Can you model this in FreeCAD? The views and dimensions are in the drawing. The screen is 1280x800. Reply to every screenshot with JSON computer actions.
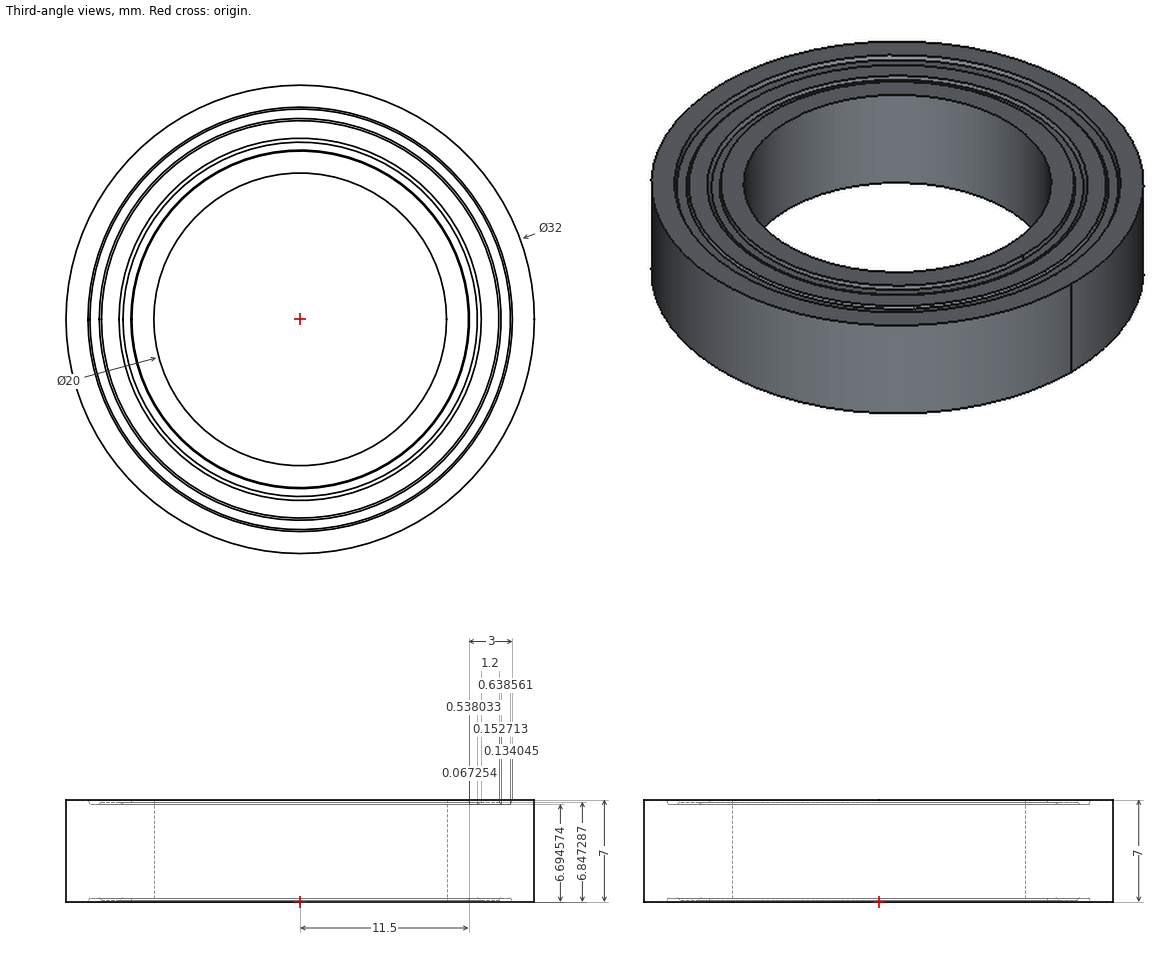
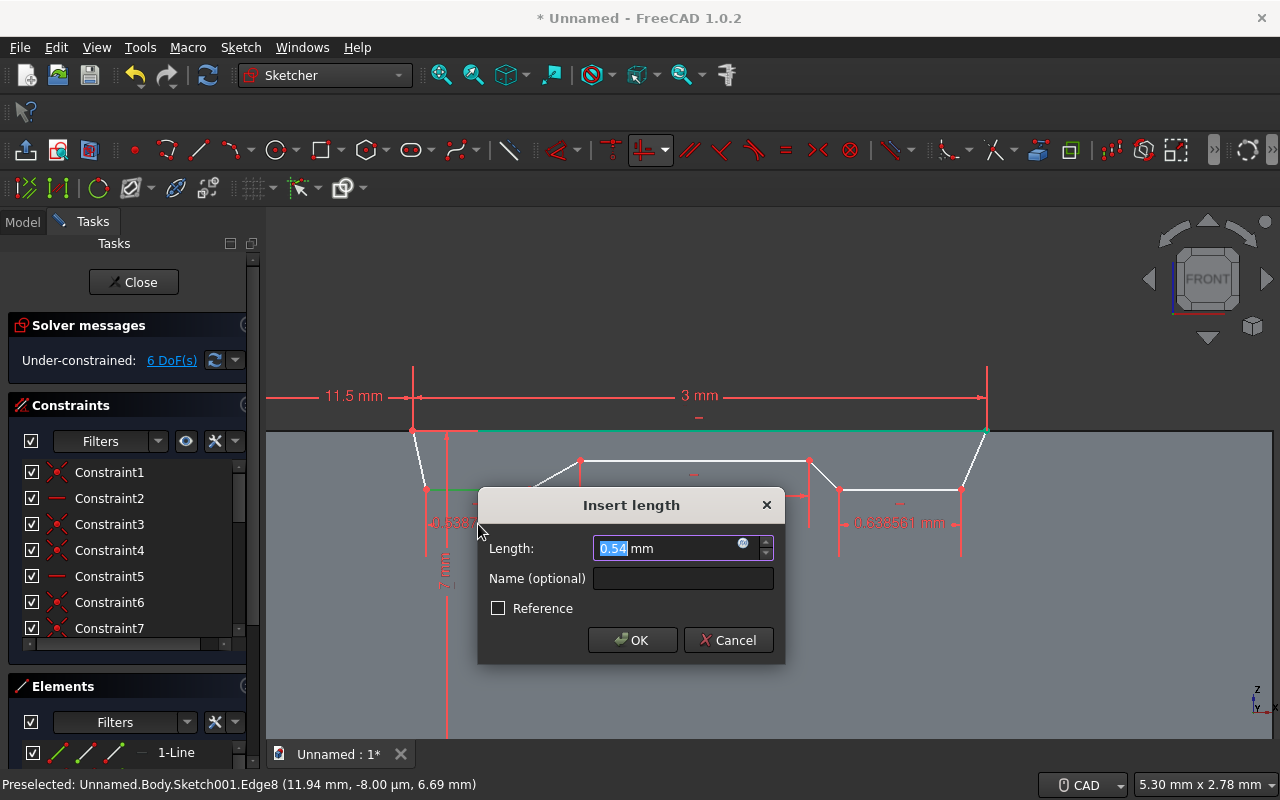
{"action": "type", "text": "0.538033"}
{"action": "key", "text": "Return"}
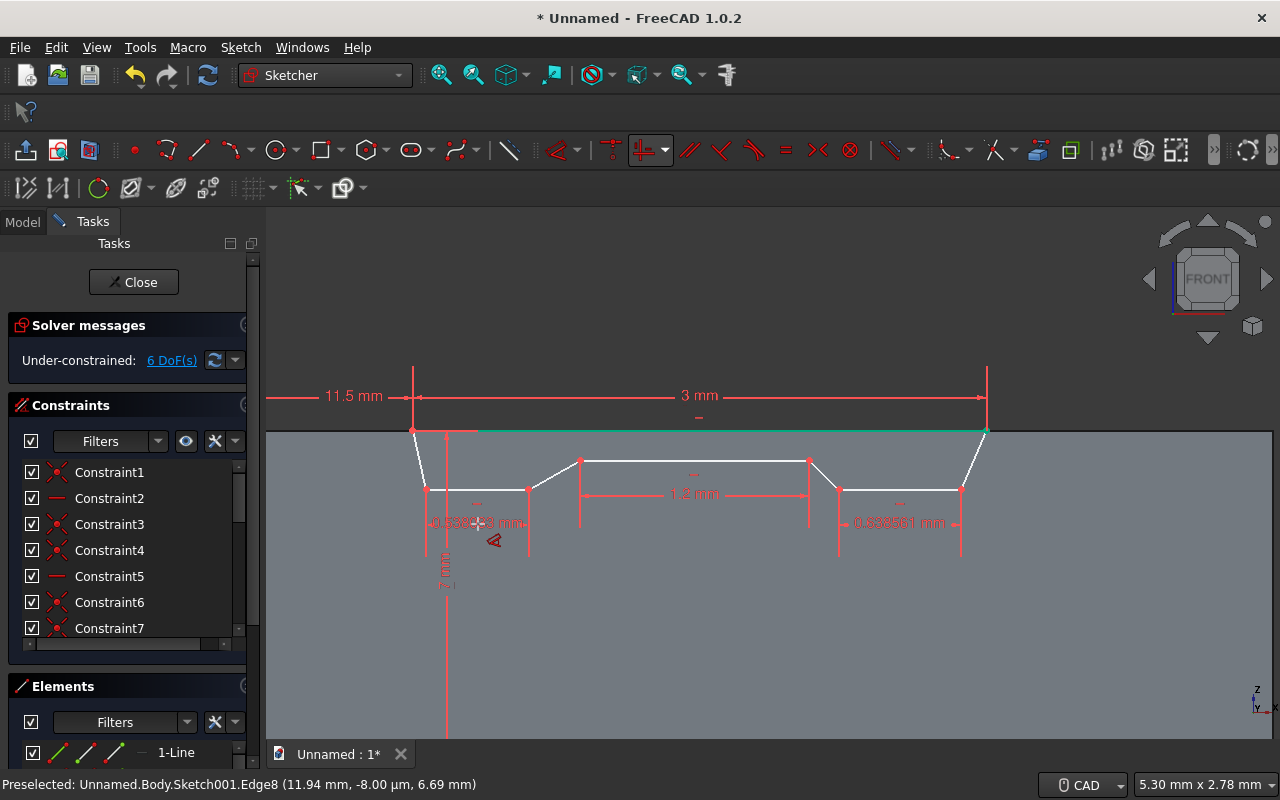
{"action": "left_click", "coordinate": [426, 490]}
{"action": "left_click", "coordinate": [460, 600]}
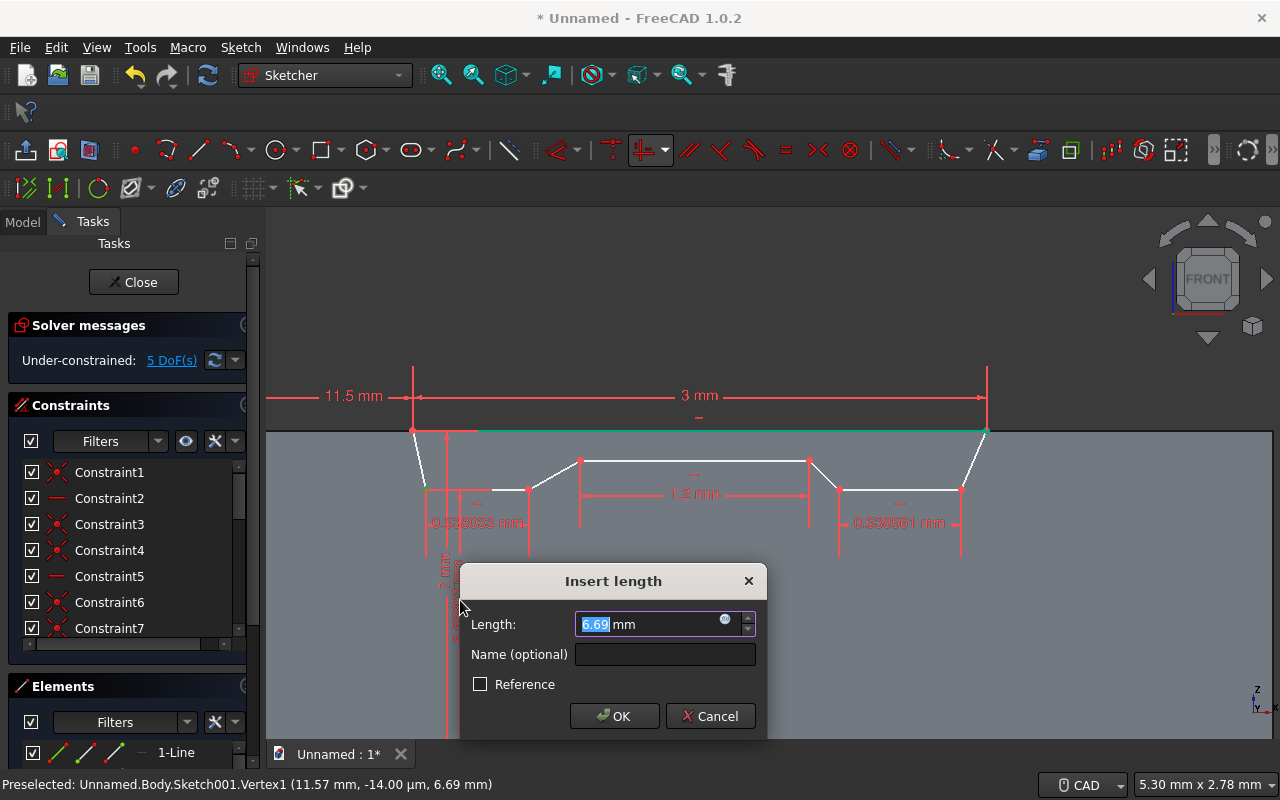
{"action": "type", "text": "6.694574"}
{"action": "key", "text": "Return"}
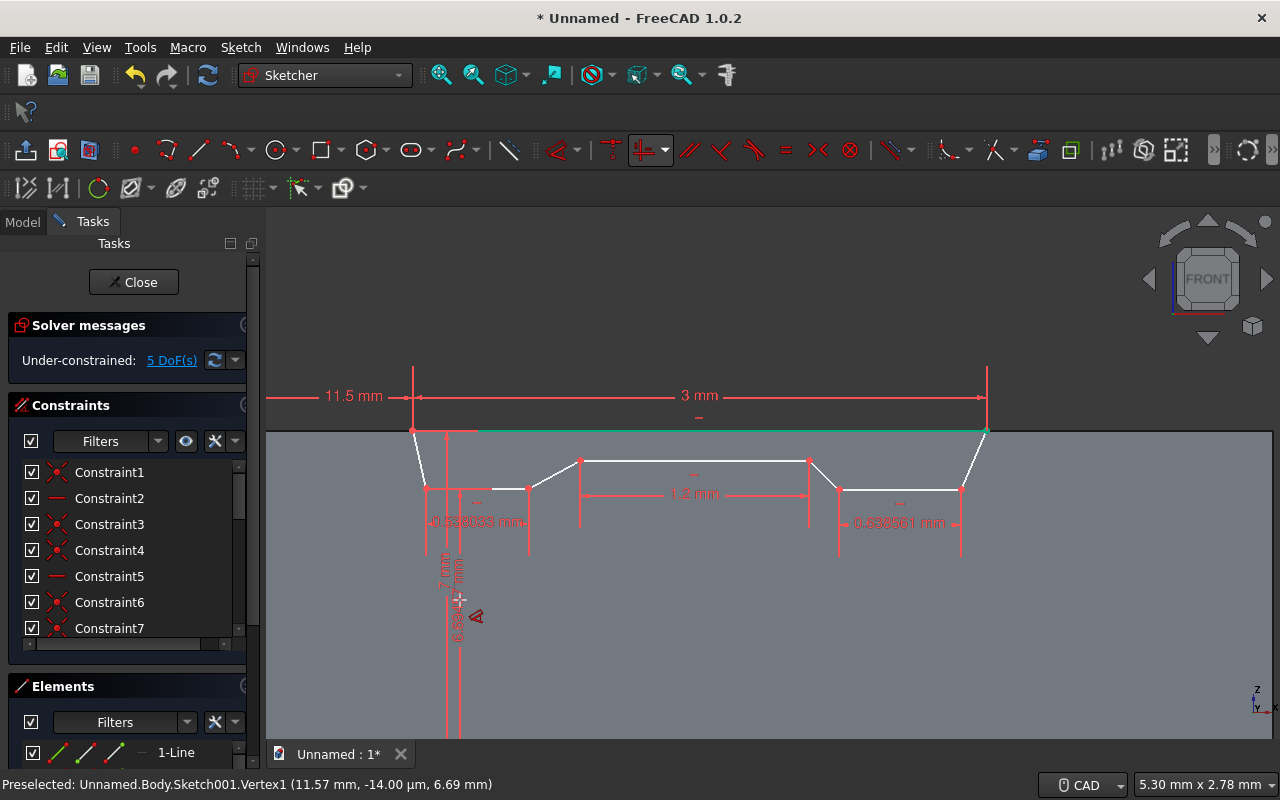
{"action": "left_click", "coordinate": [961, 490]}
{"action": "left_click", "coordinate": [995, 600]}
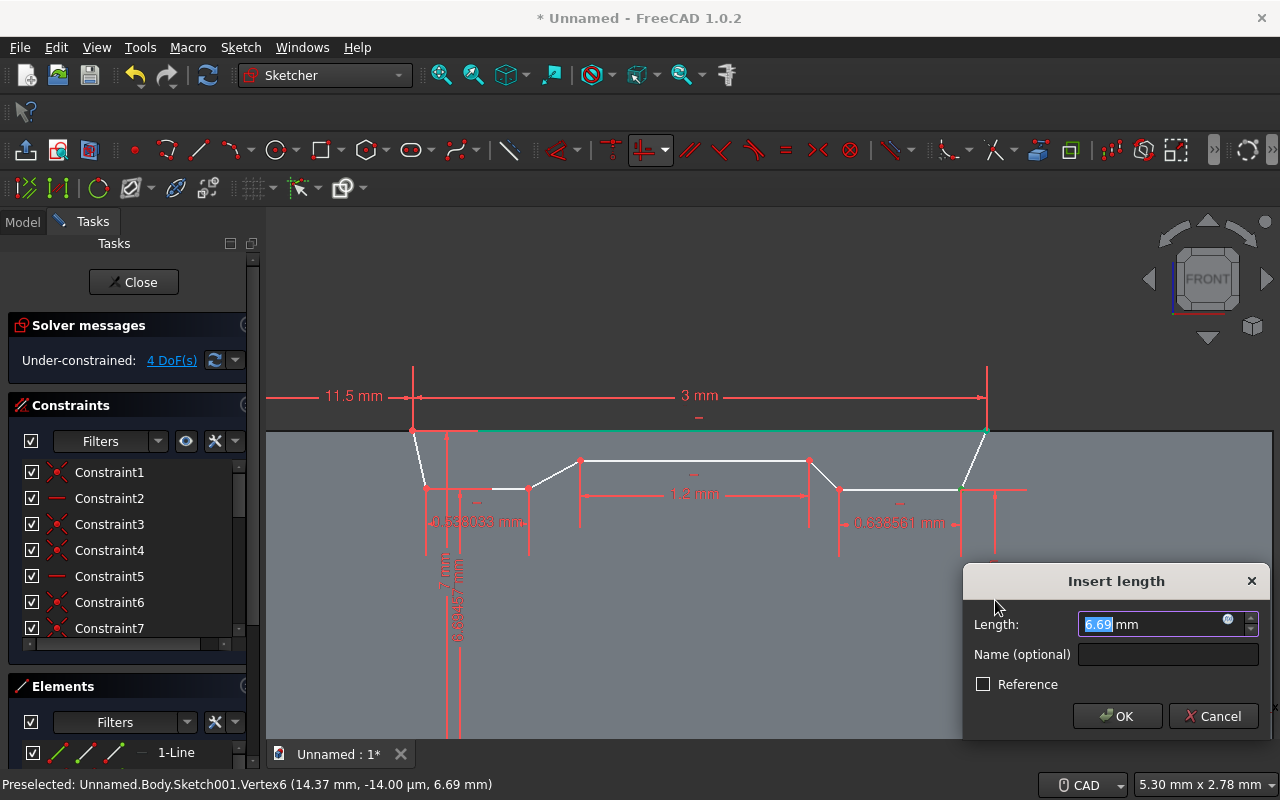
{"action": "type", "text": "6.694574"}
{"action": "key", "text": "Return"}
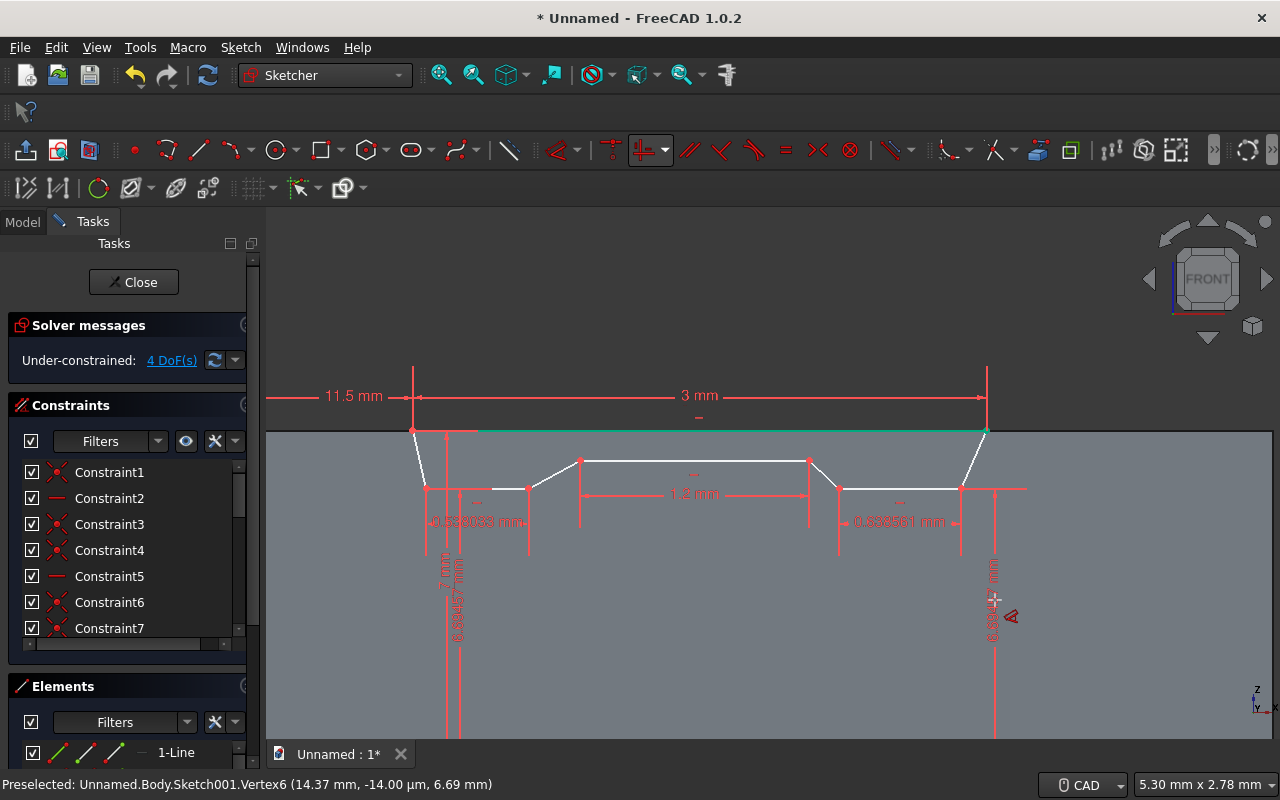
{"action": "left_click", "coordinate": [809, 461]}
{"action": "left_click", "coordinate": [843, 586]}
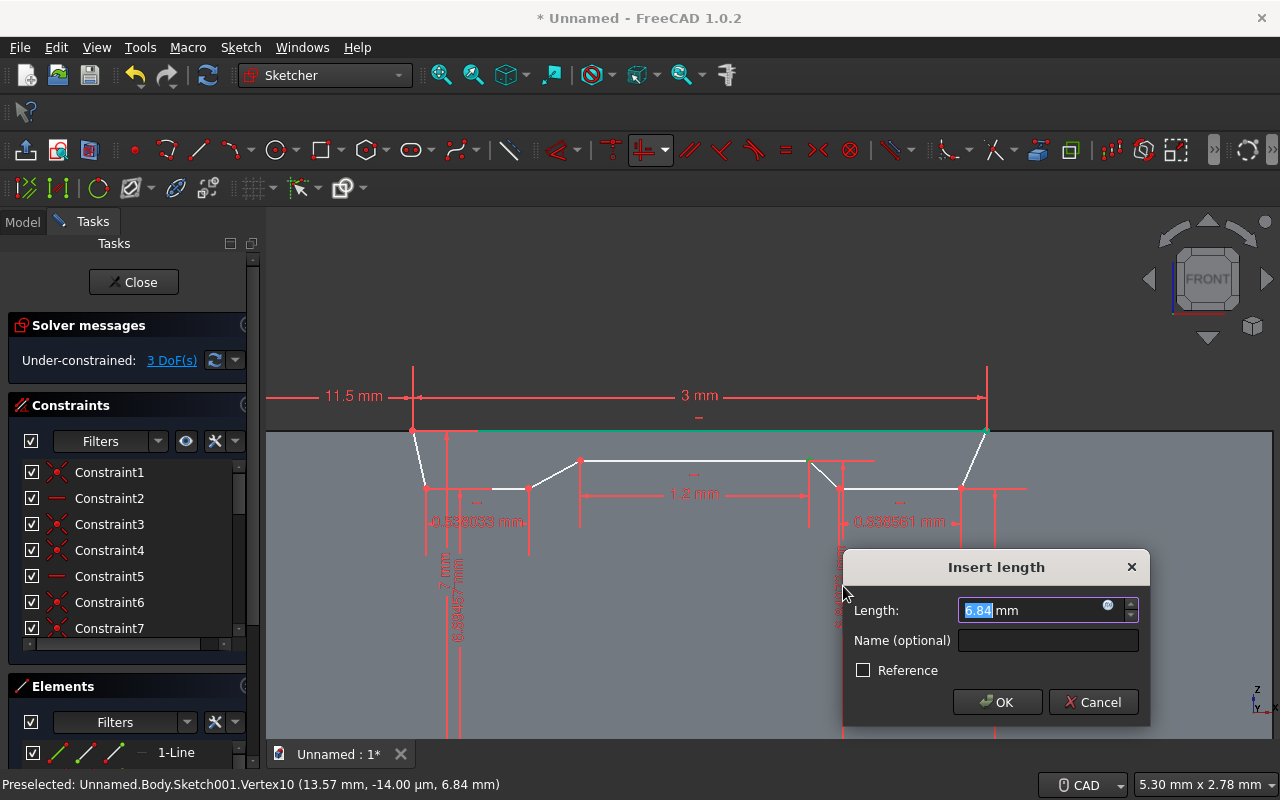
{"action": "type", "text": "6.847287"}
{"action": "key", "text": "Return"}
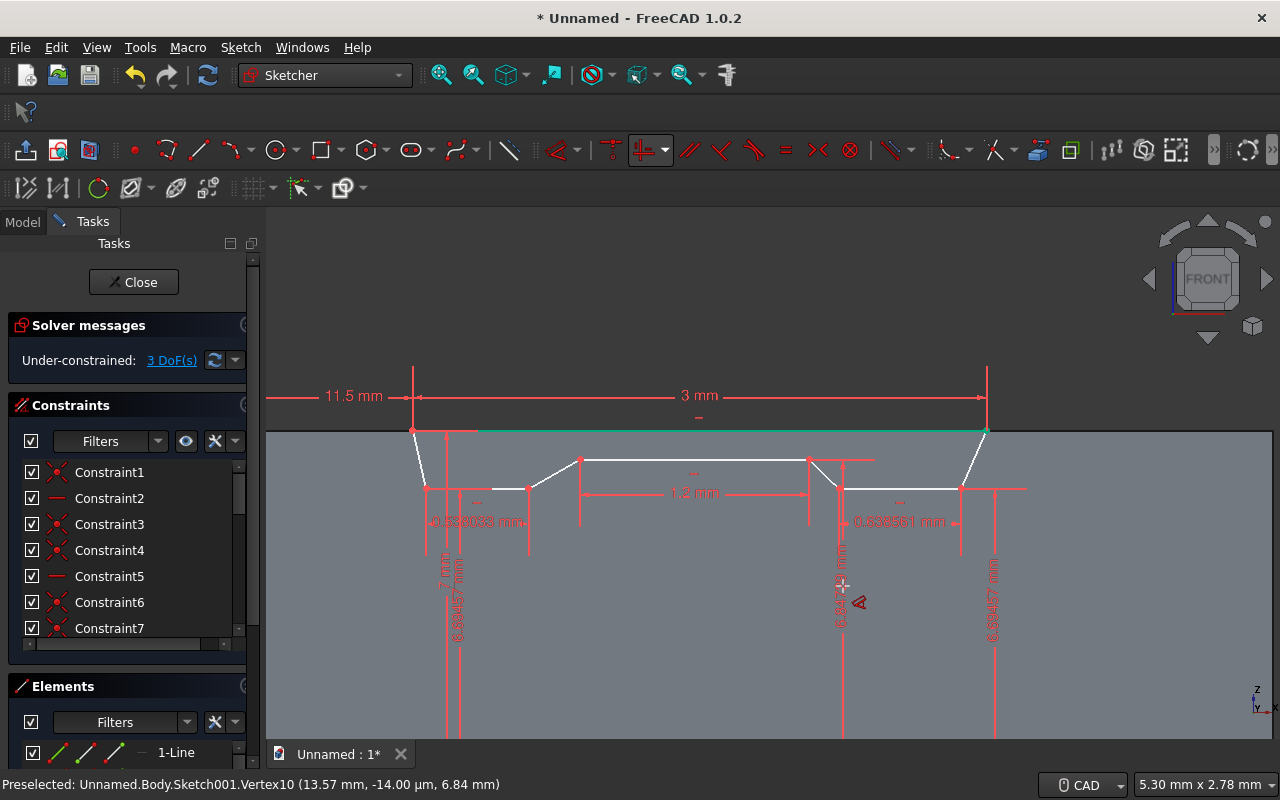
{"action": "scroll", "coordinate": [422, 471], "scroll_direction": "up", "scroll_amount": 6}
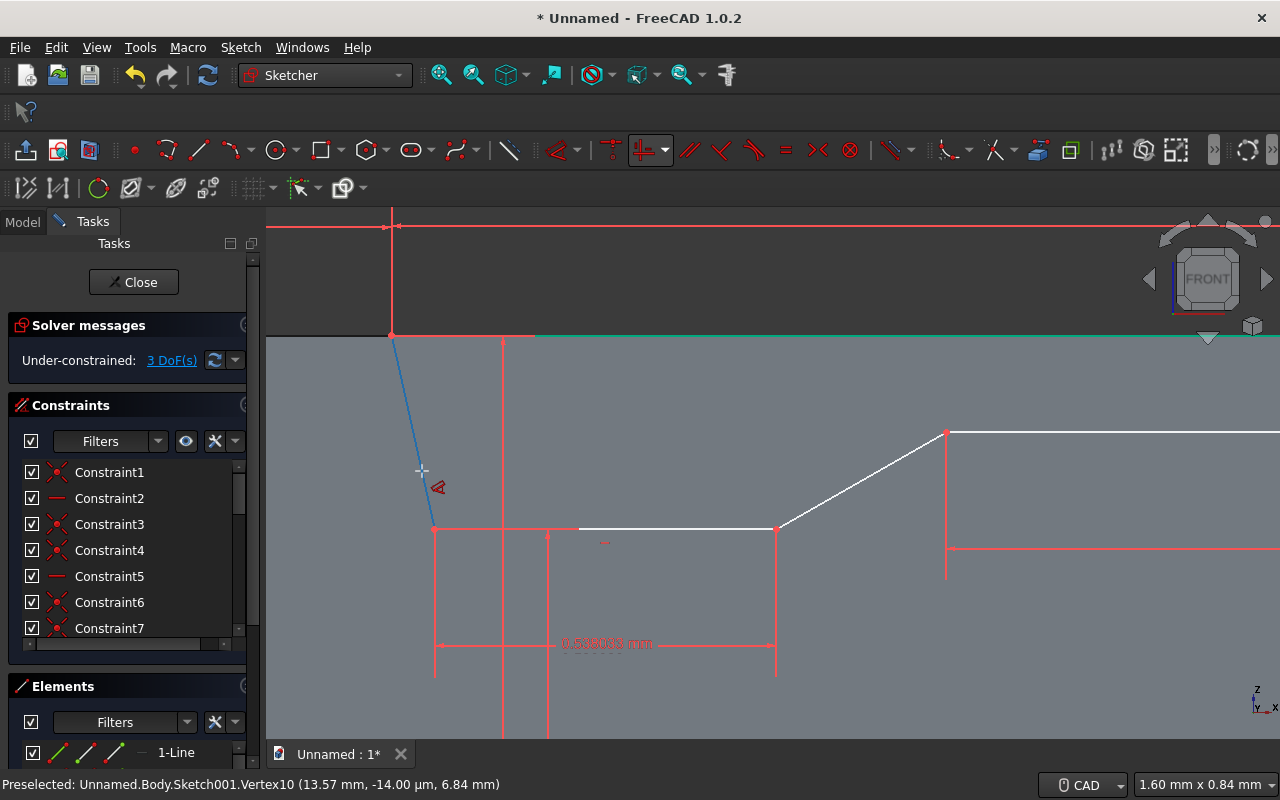
{"action": "left_click", "coordinate": [422, 471]}
{"action": "left_click", "coordinate": [413, 302]}